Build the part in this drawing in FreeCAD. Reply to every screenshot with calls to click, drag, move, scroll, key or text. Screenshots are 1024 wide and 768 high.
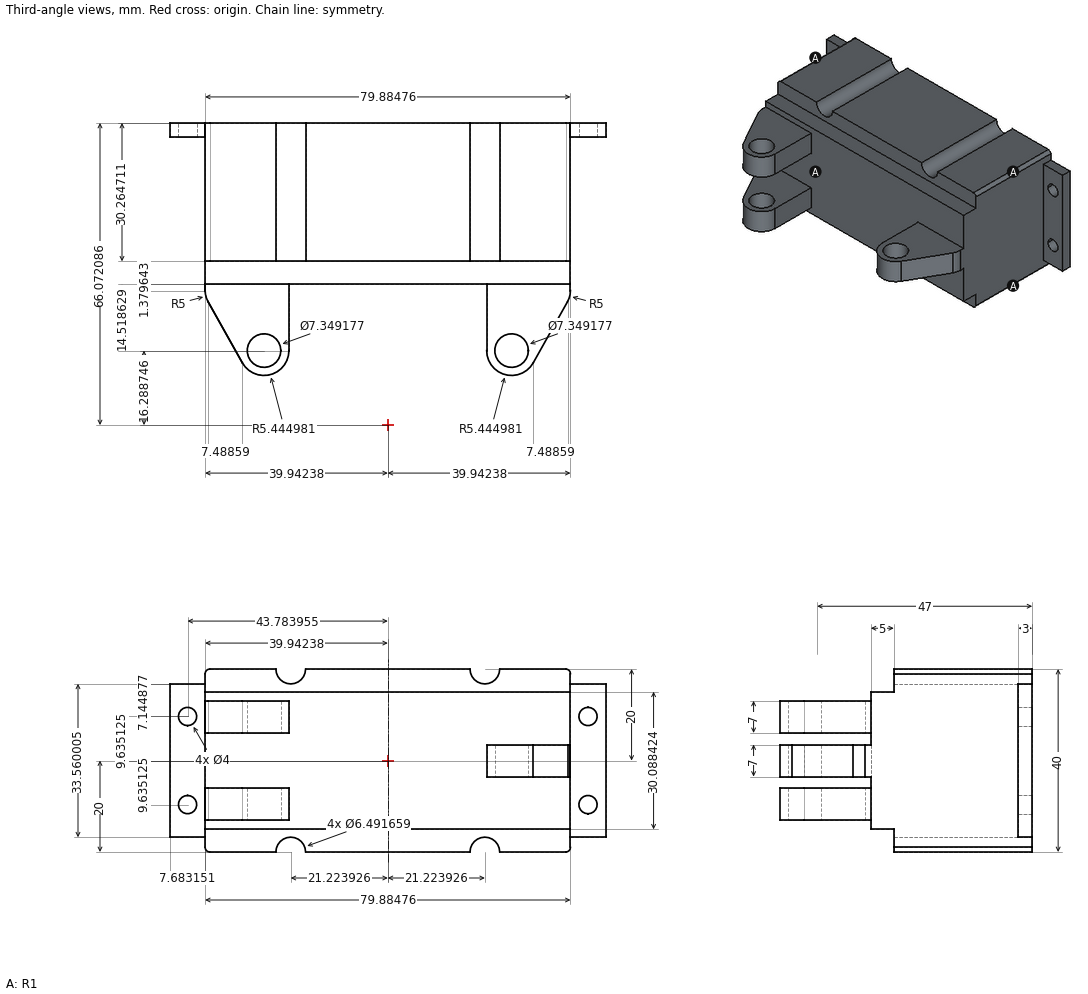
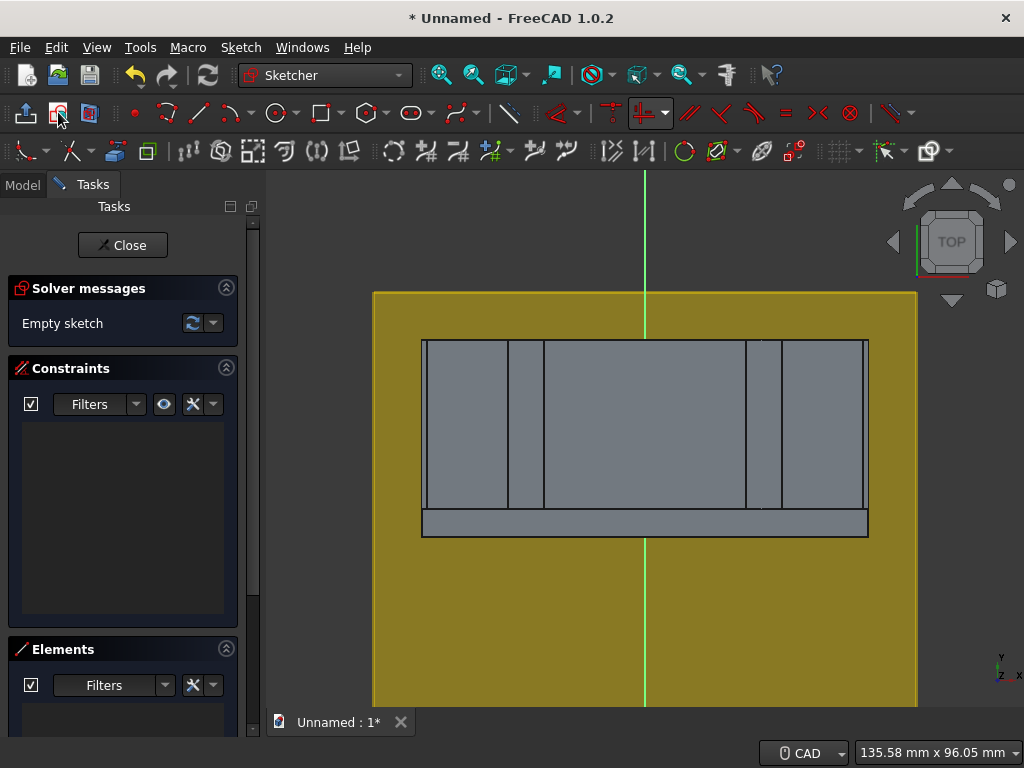
click(90, 114)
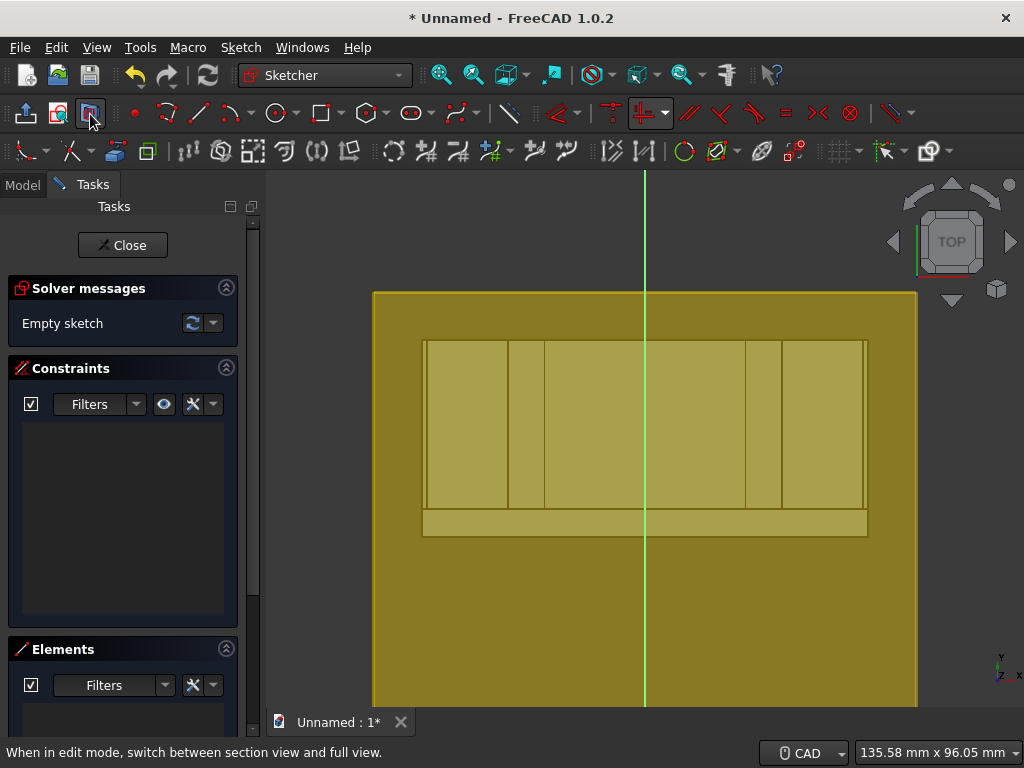
scroll(576, 438, down, 5)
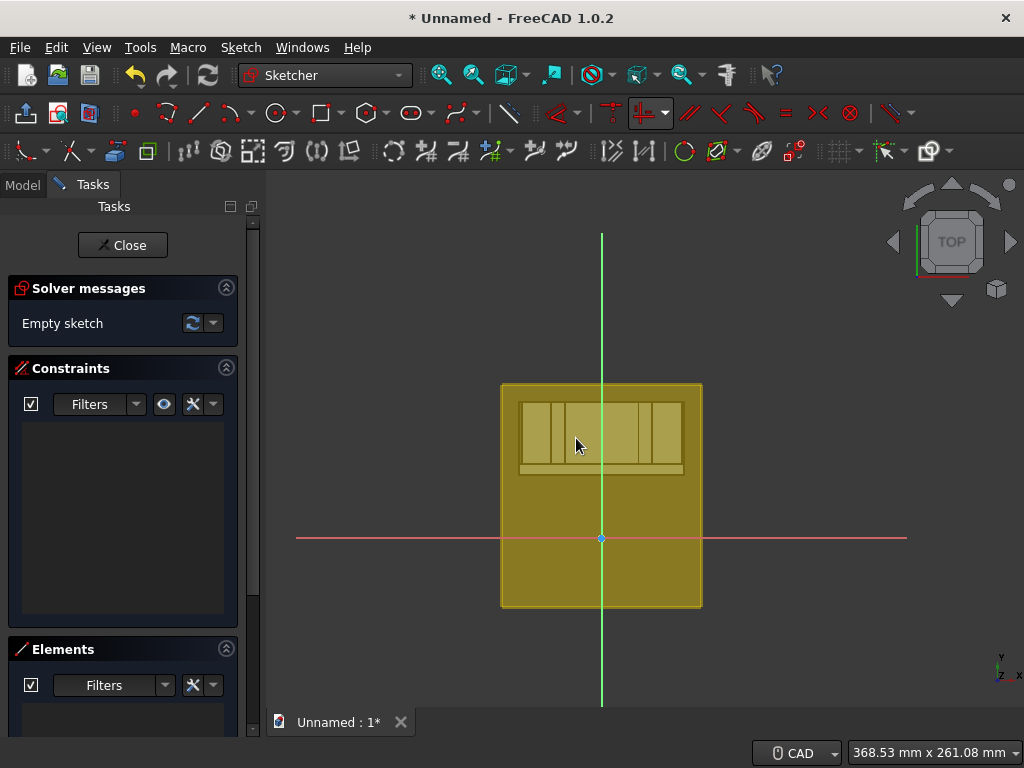
scroll(557, 524, up, 8)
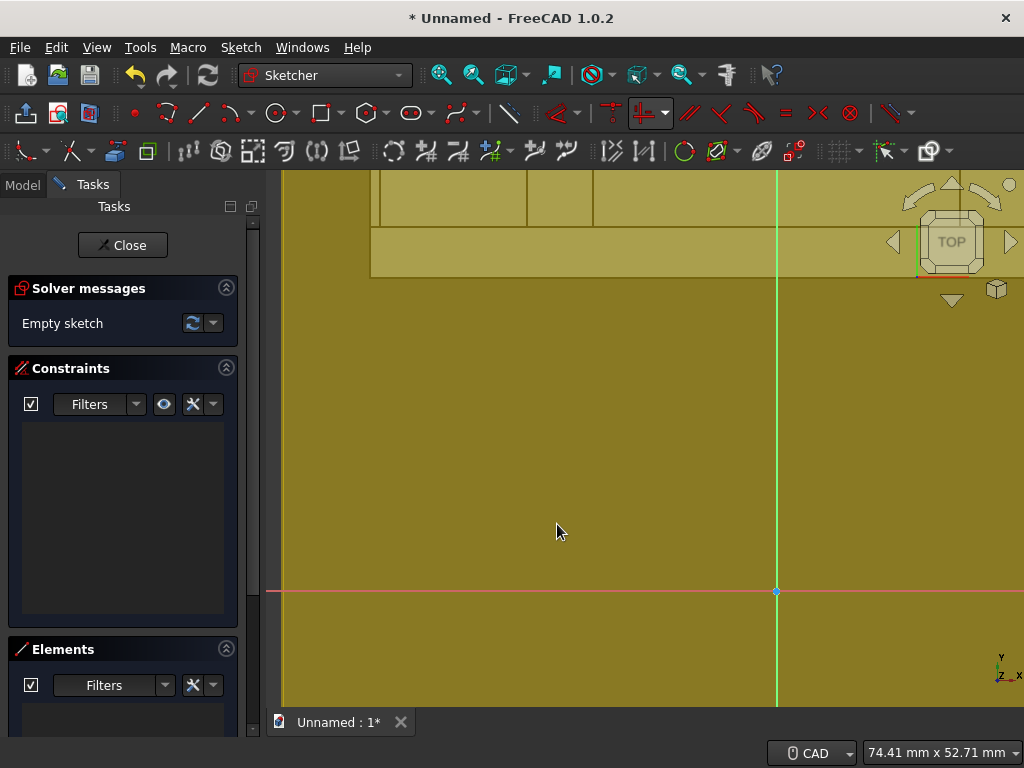
click(200, 114)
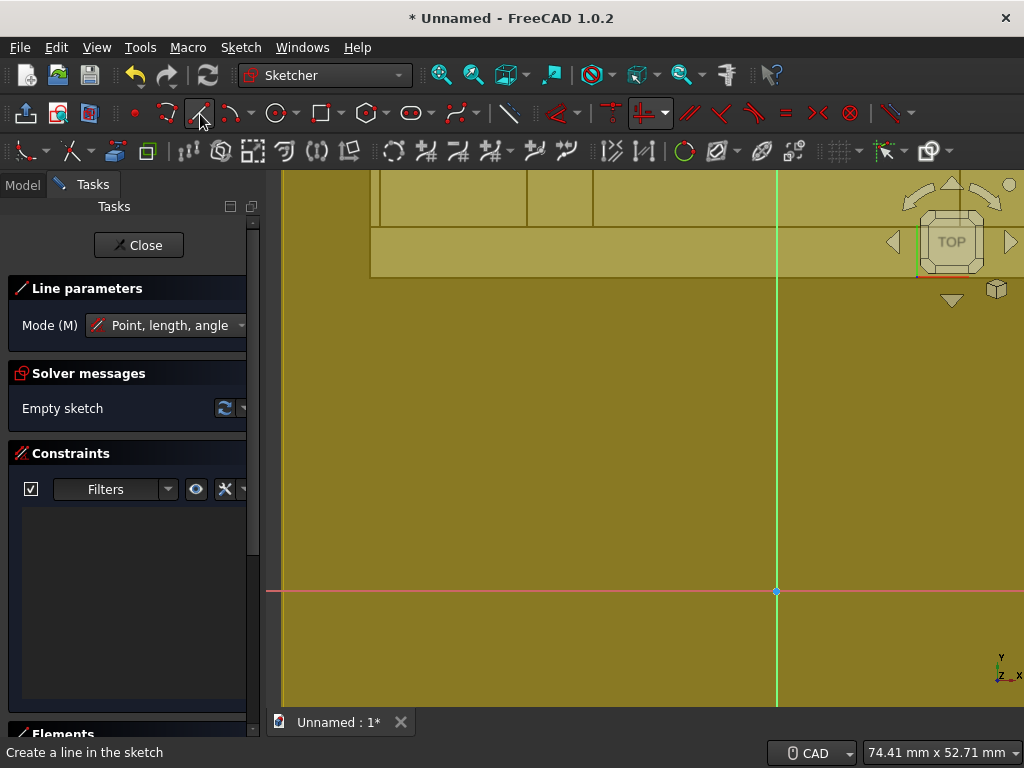
click(376, 316)
click(452, 453)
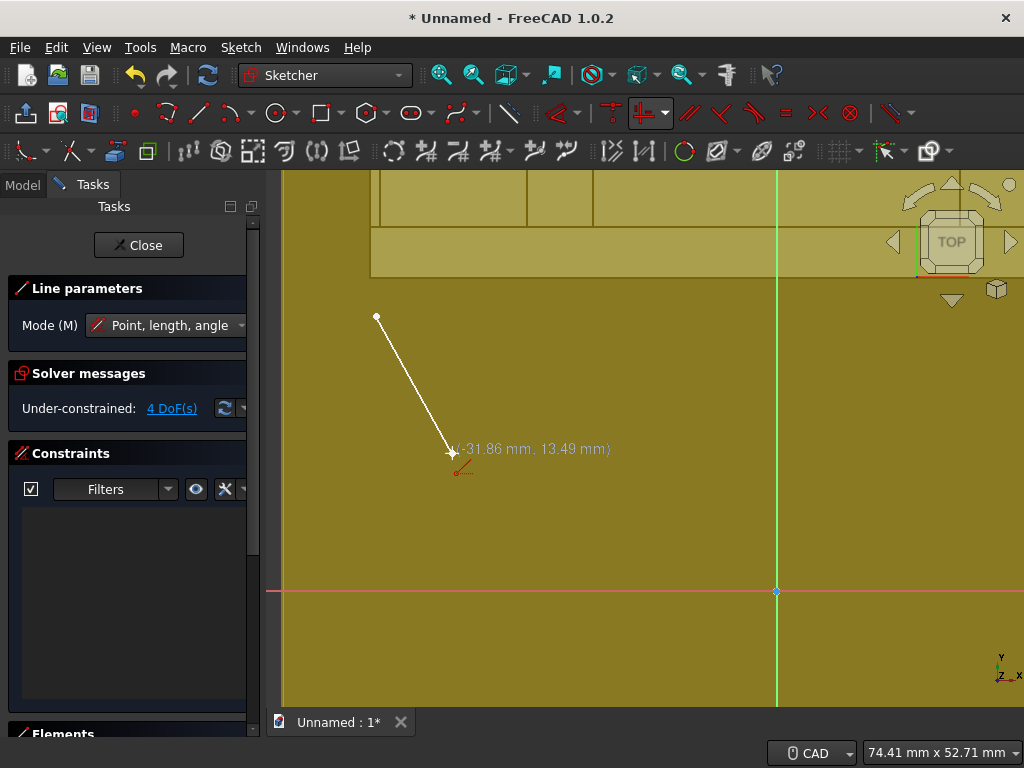
click(168, 114)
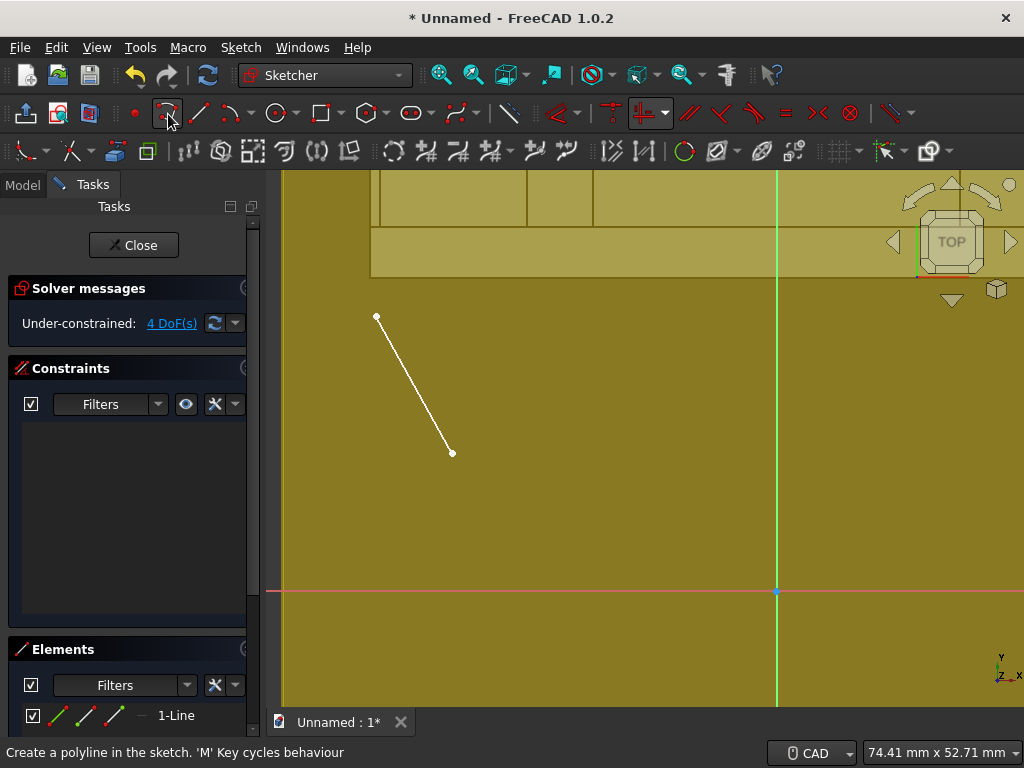
click(556, 425)
click(556, 278)
click(370, 278)
click(370, 292)
right_click(370, 292)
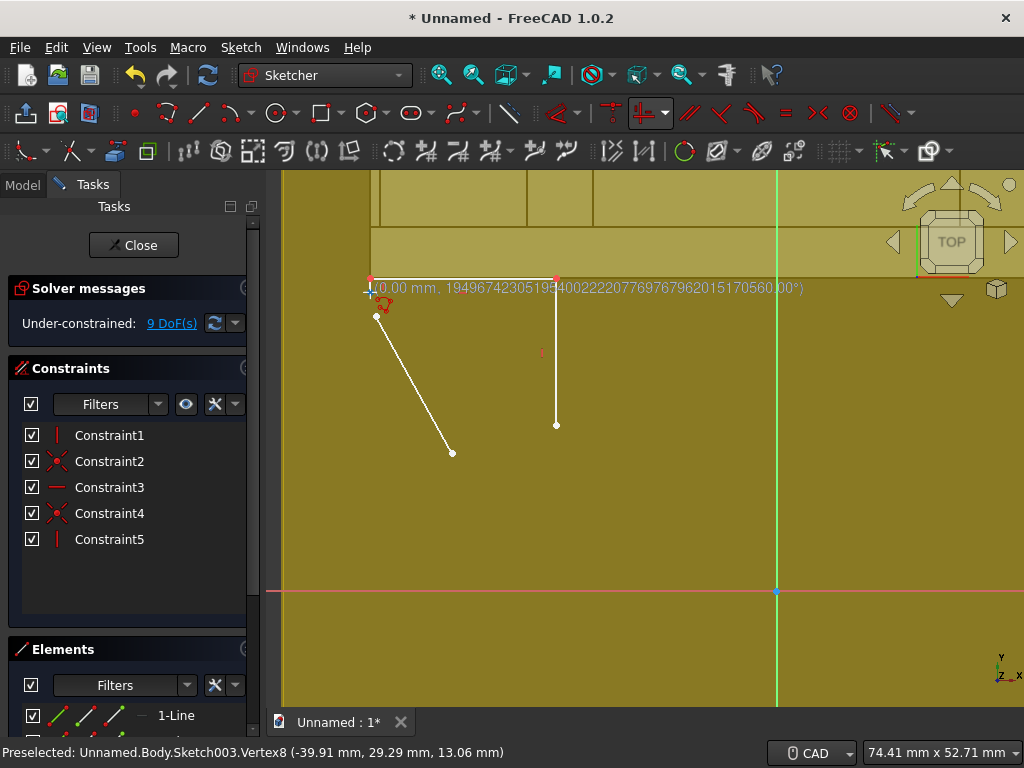
key(g)
key(3)
key(a)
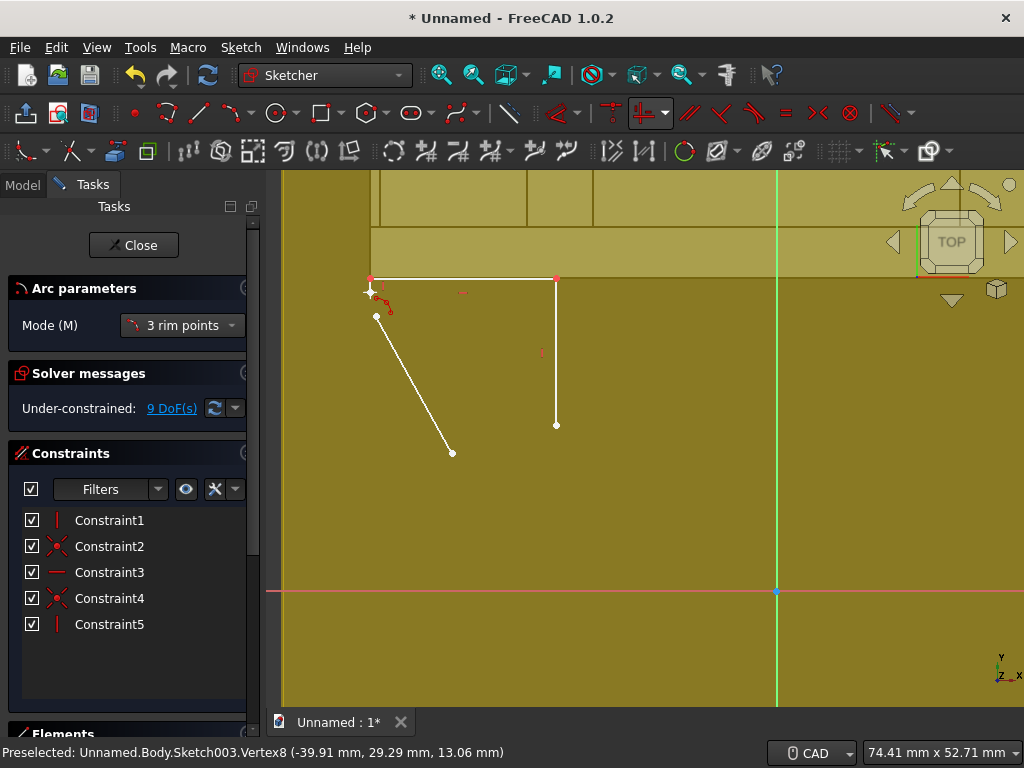
click(452, 454)
click(556, 426)
click(515, 479)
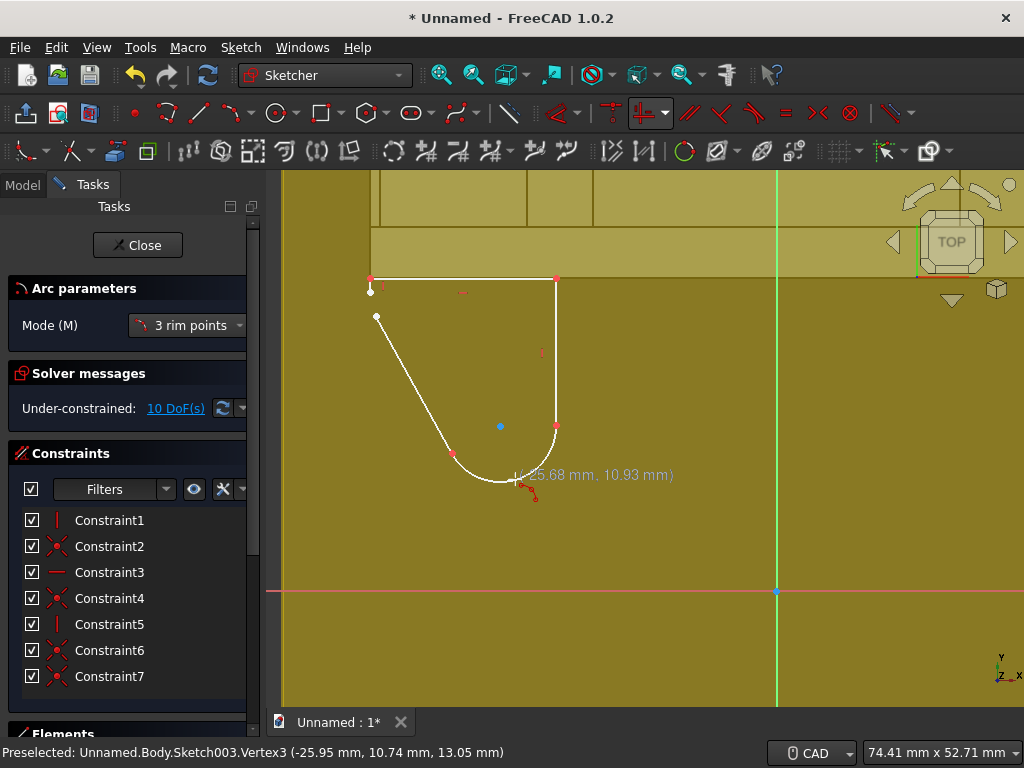
scroll(370, 292, up, 5)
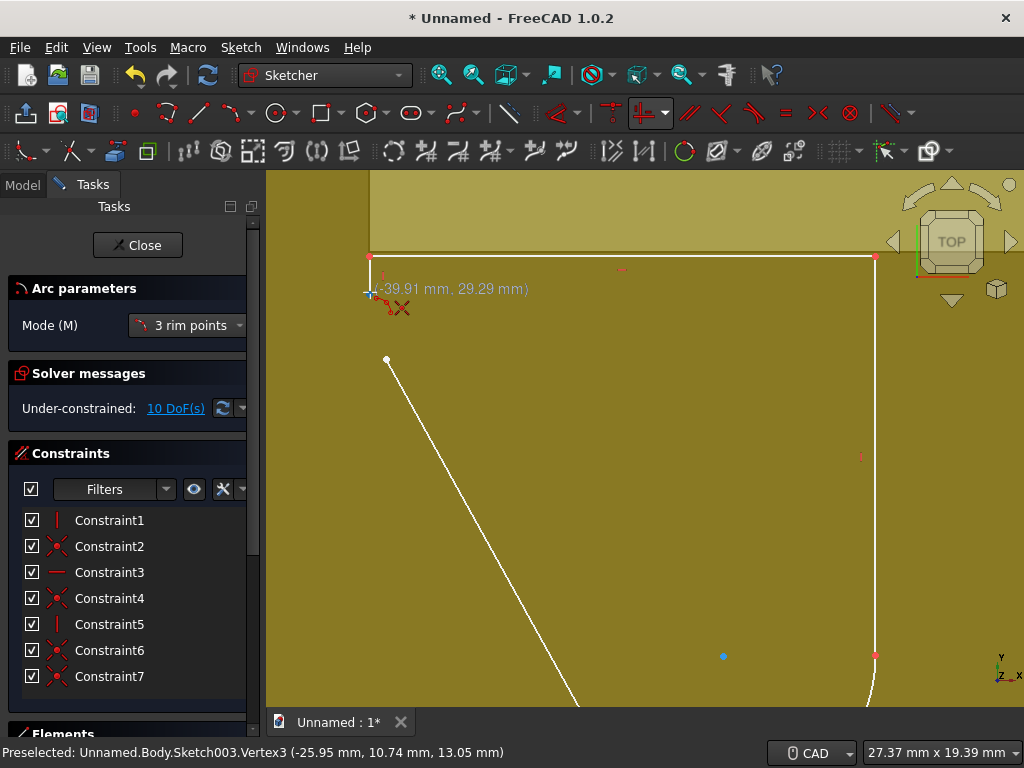
click(370, 294)
click(386, 360)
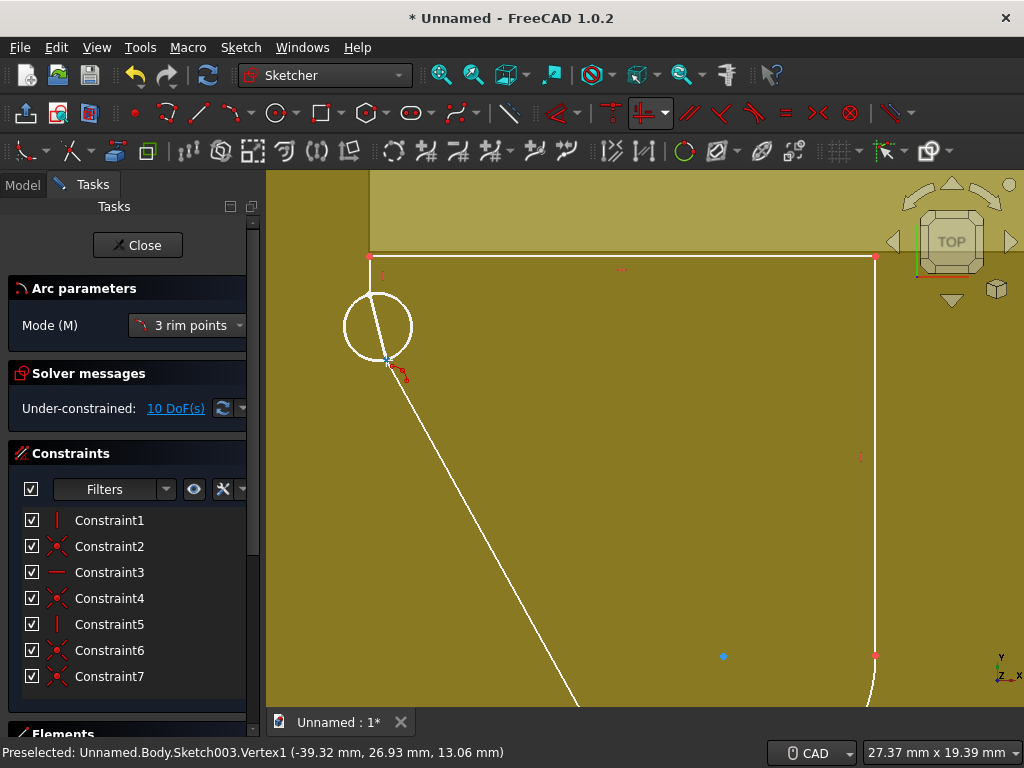
scroll(373, 325, up, 7)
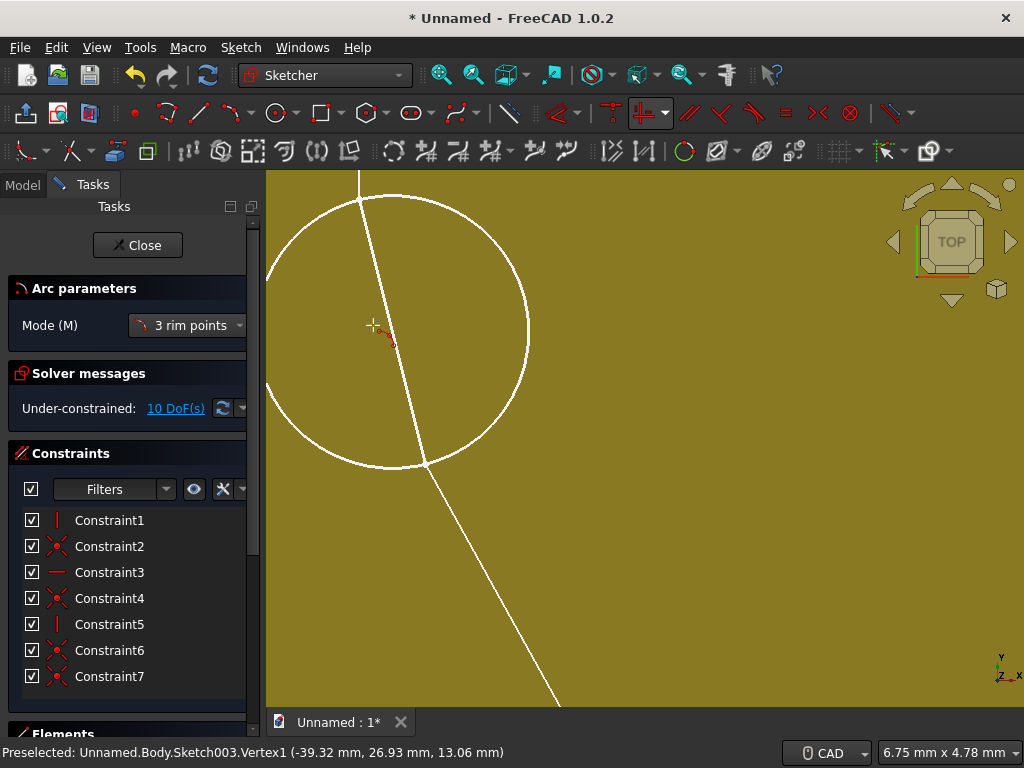
click(374, 326)